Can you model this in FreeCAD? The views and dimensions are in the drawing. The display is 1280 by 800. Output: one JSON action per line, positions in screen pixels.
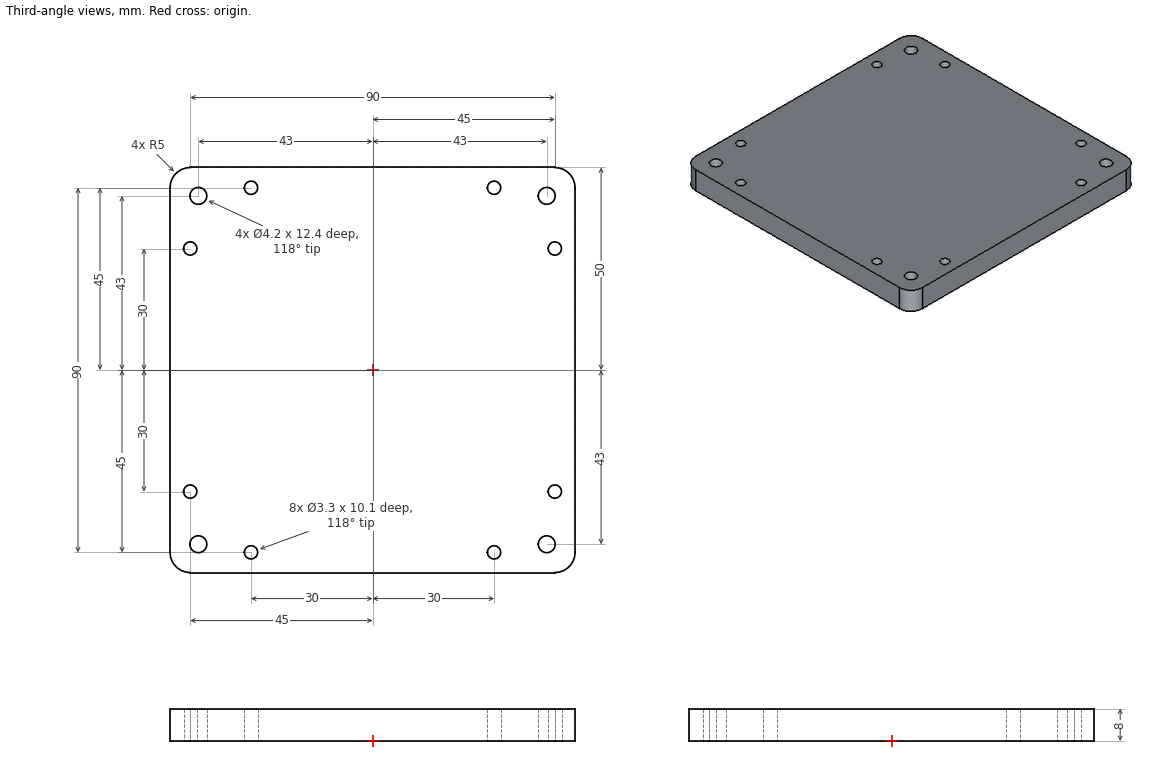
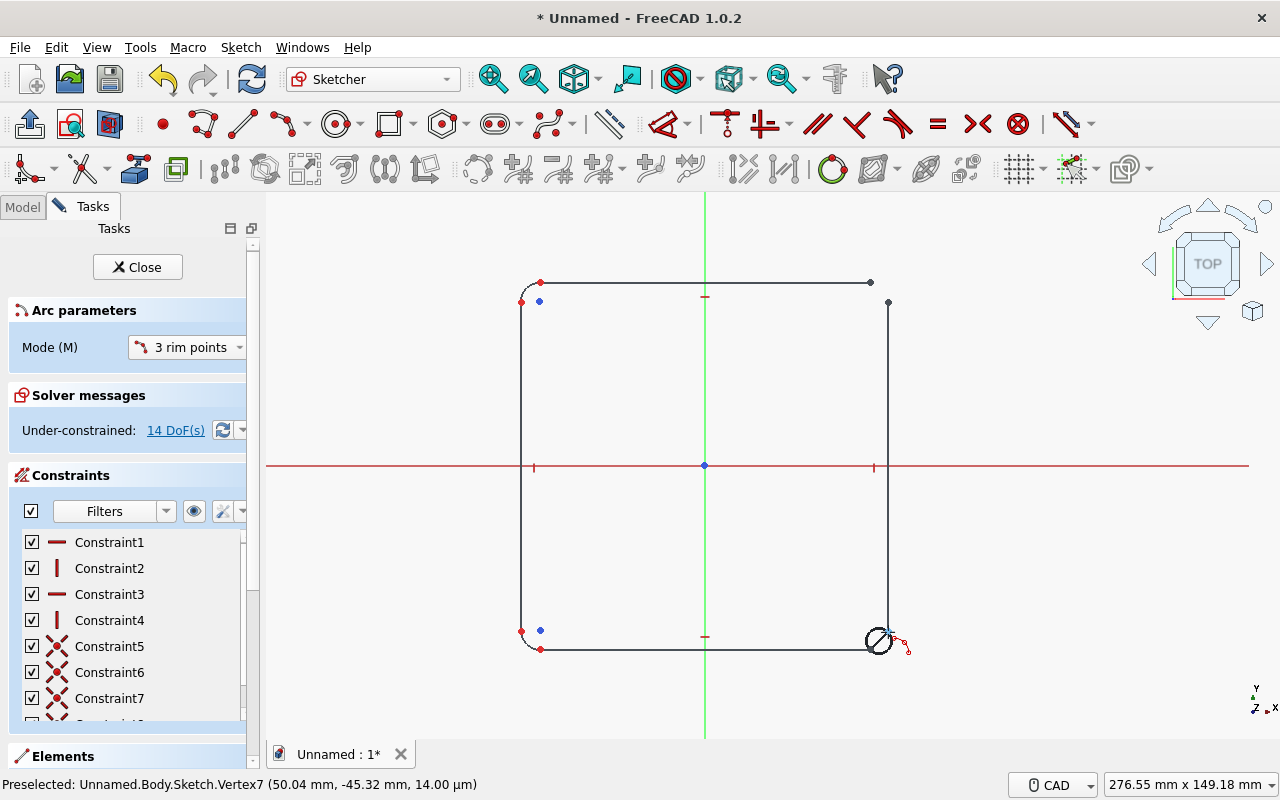
{"action": "scroll", "coordinate": [882, 644], "scroll_direction": "up", "scroll_amount": 6}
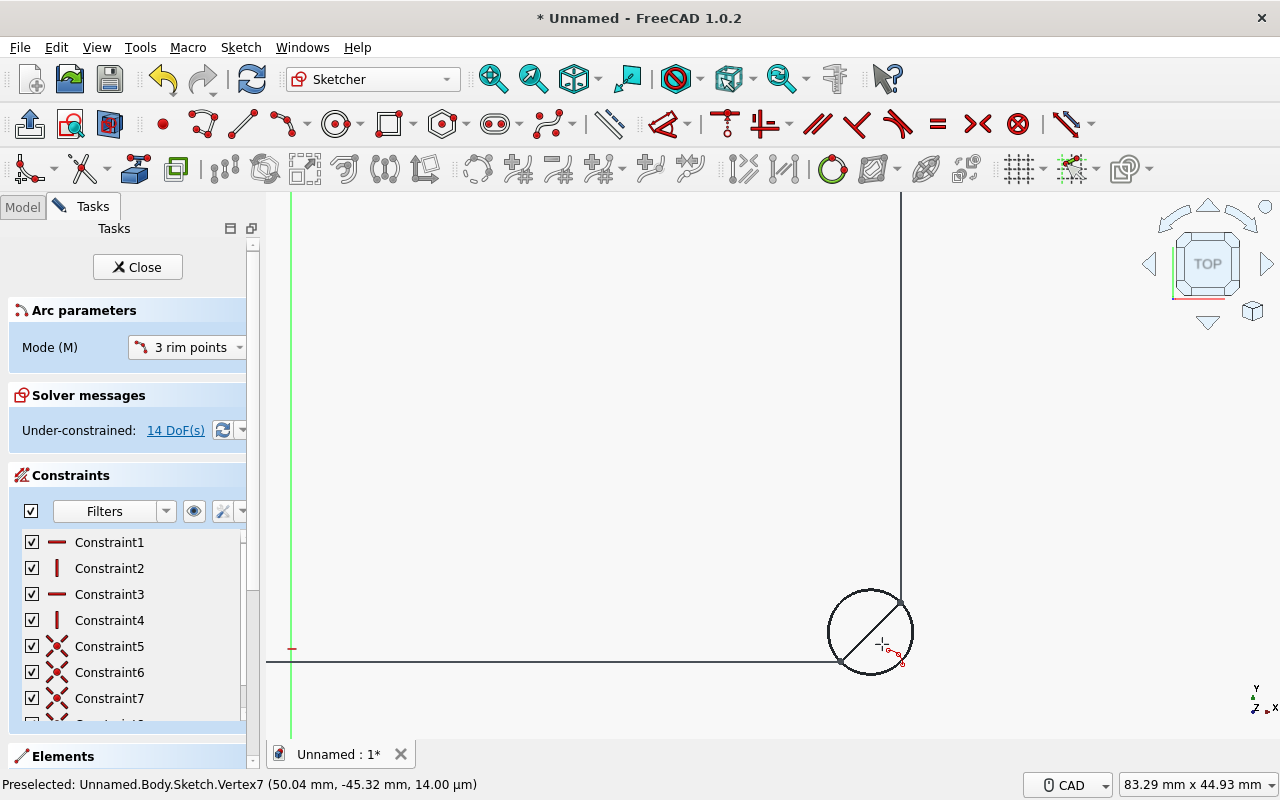
{"action": "left_click", "coordinate": [882, 641]}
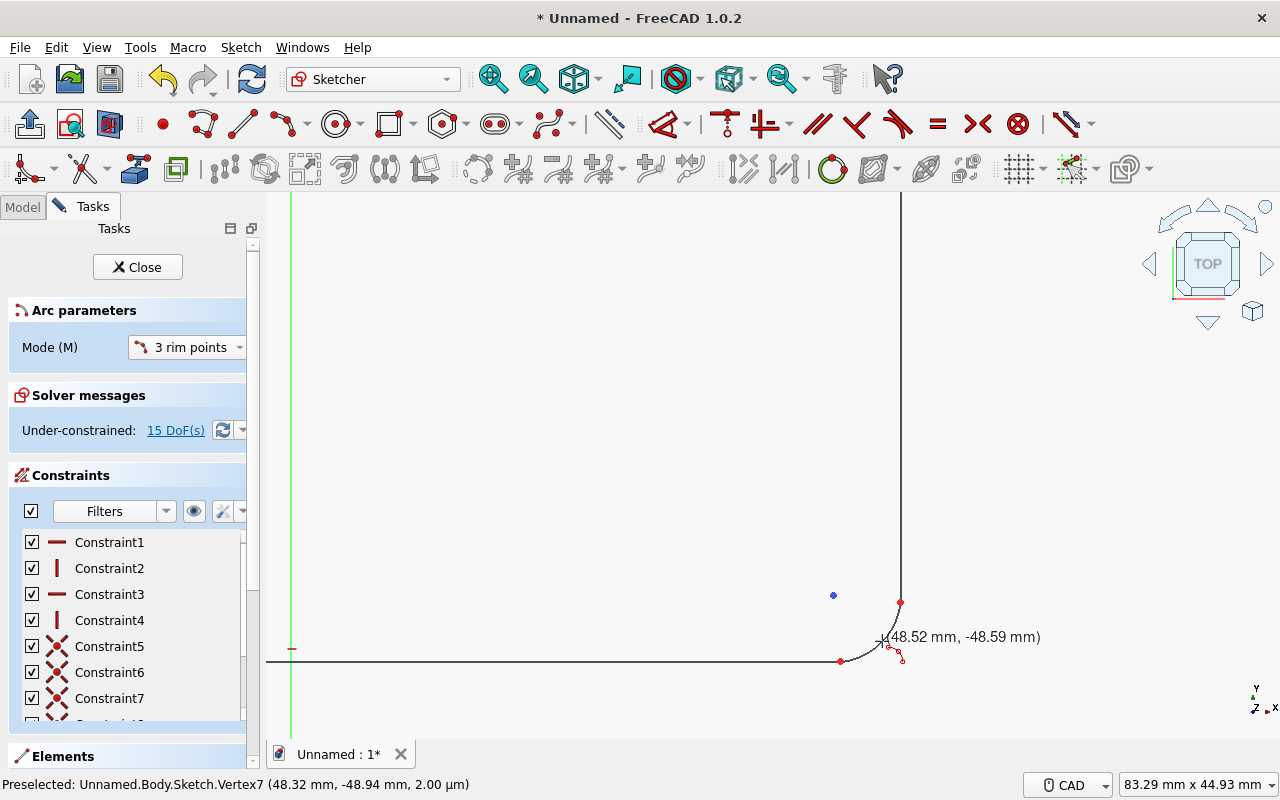
{"action": "scroll", "coordinate": [883, 644], "scroll_direction": "down", "scroll_amount": 6}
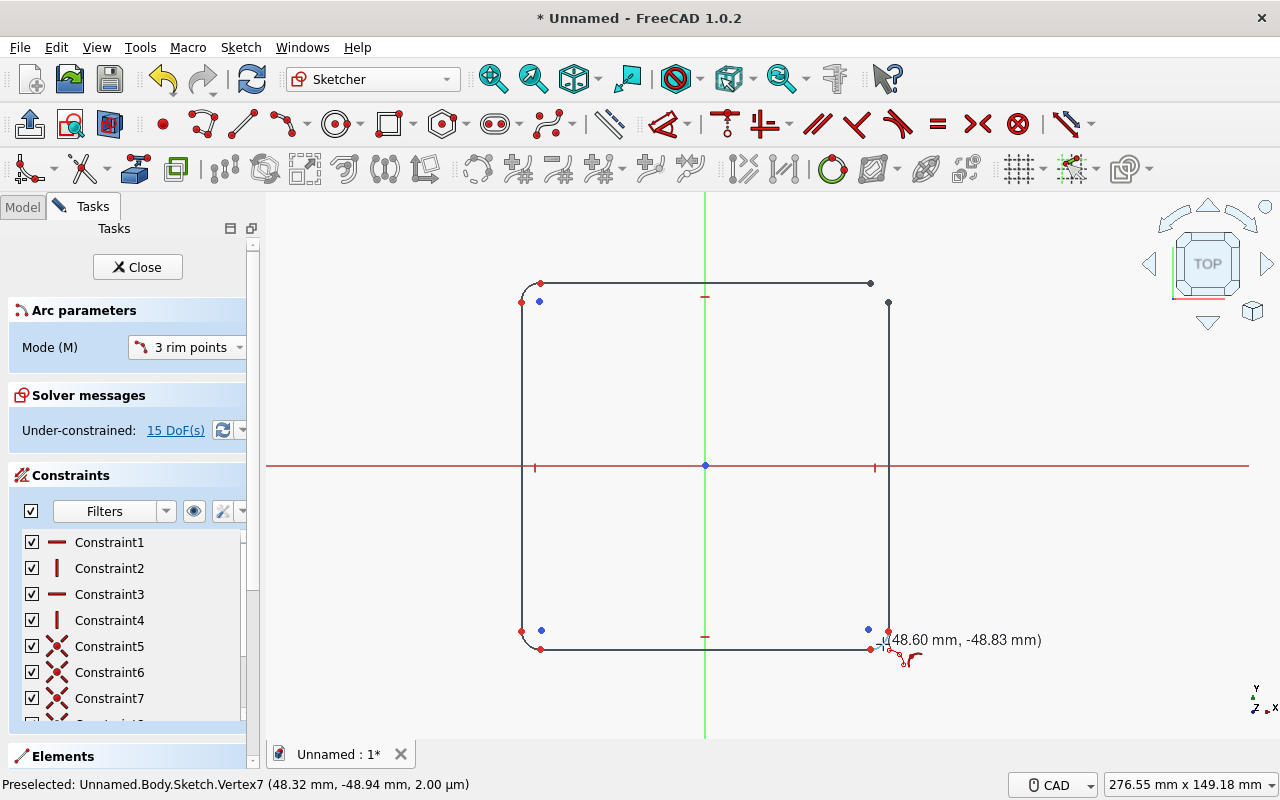
{"action": "left_click", "coordinate": [889, 302]}
{"action": "left_click", "coordinate": [871, 283]}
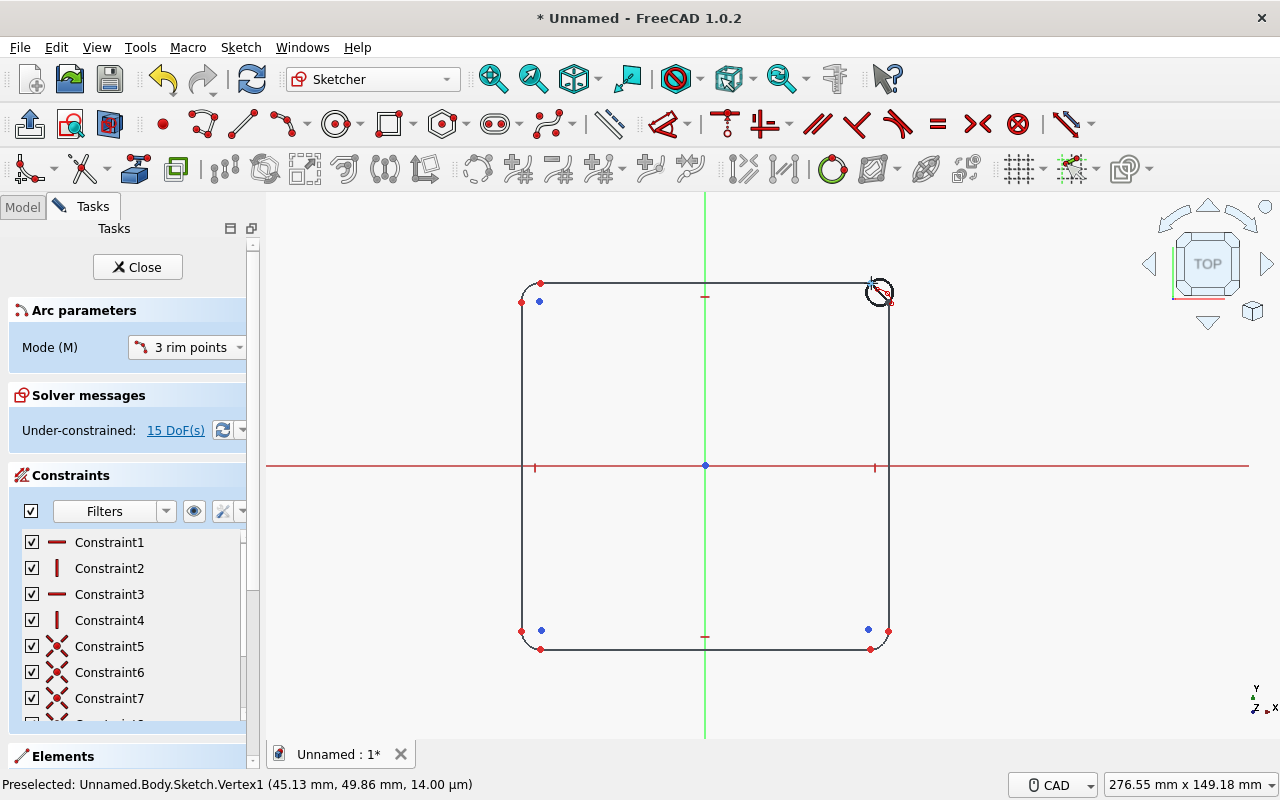
{"action": "scroll", "coordinate": [883, 288], "scroll_direction": "up", "scroll_amount": 6}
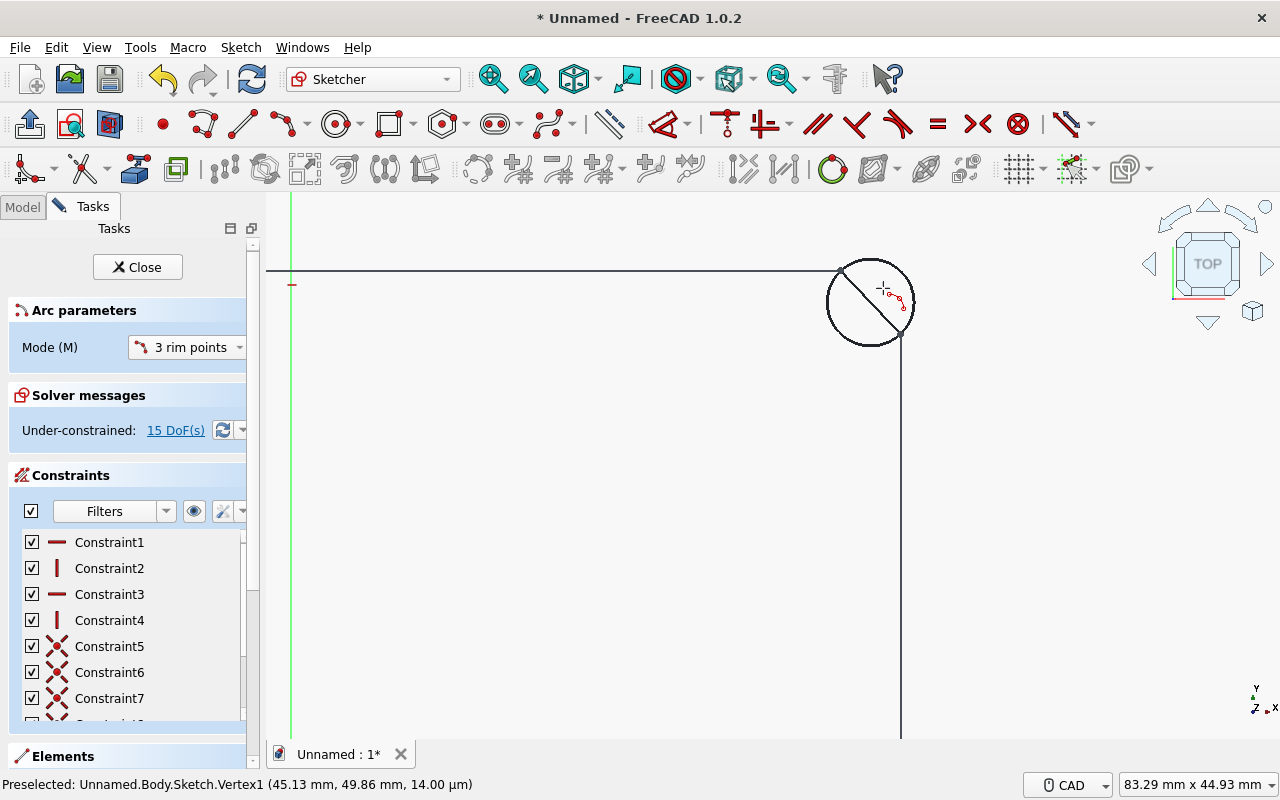
{"action": "left_click", "coordinate": [882, 287]}
{"action": "key", "text": "Escape"}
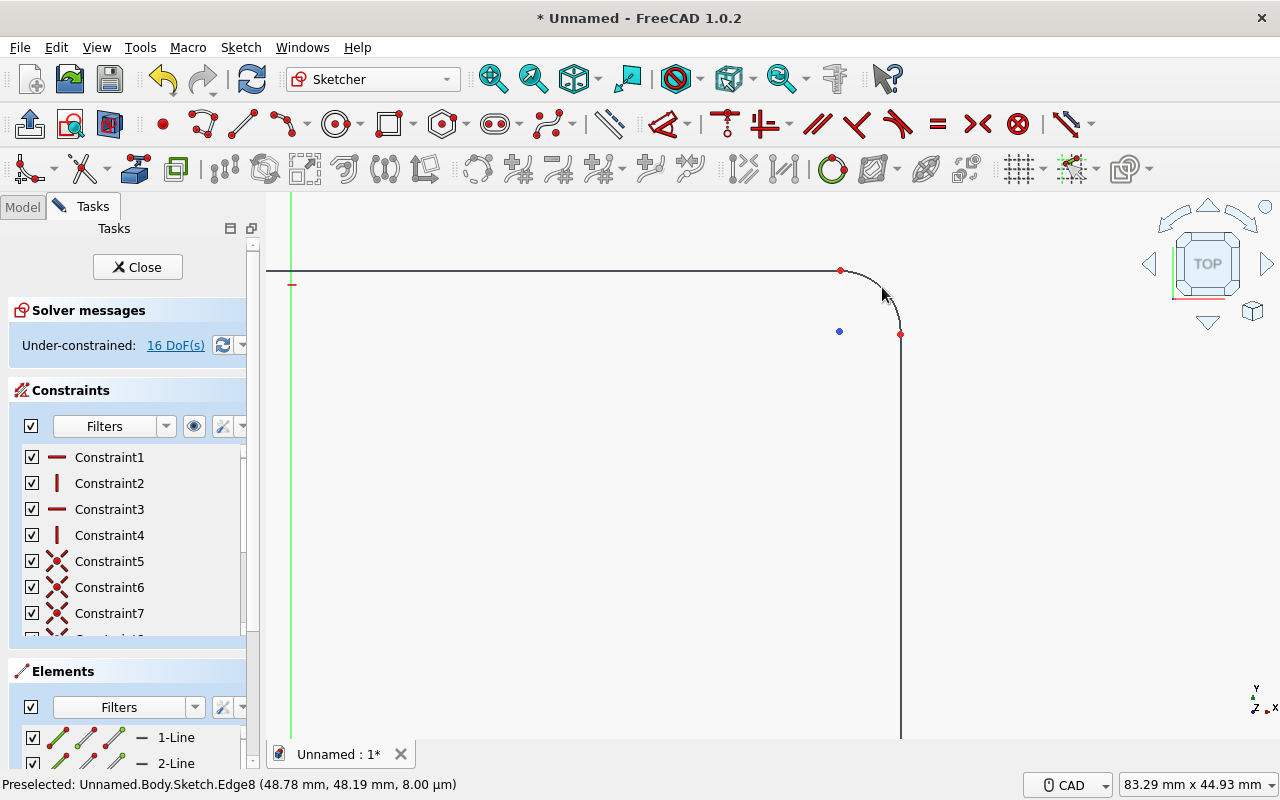
{"action": "left_click", "coordinate": [512, 271]}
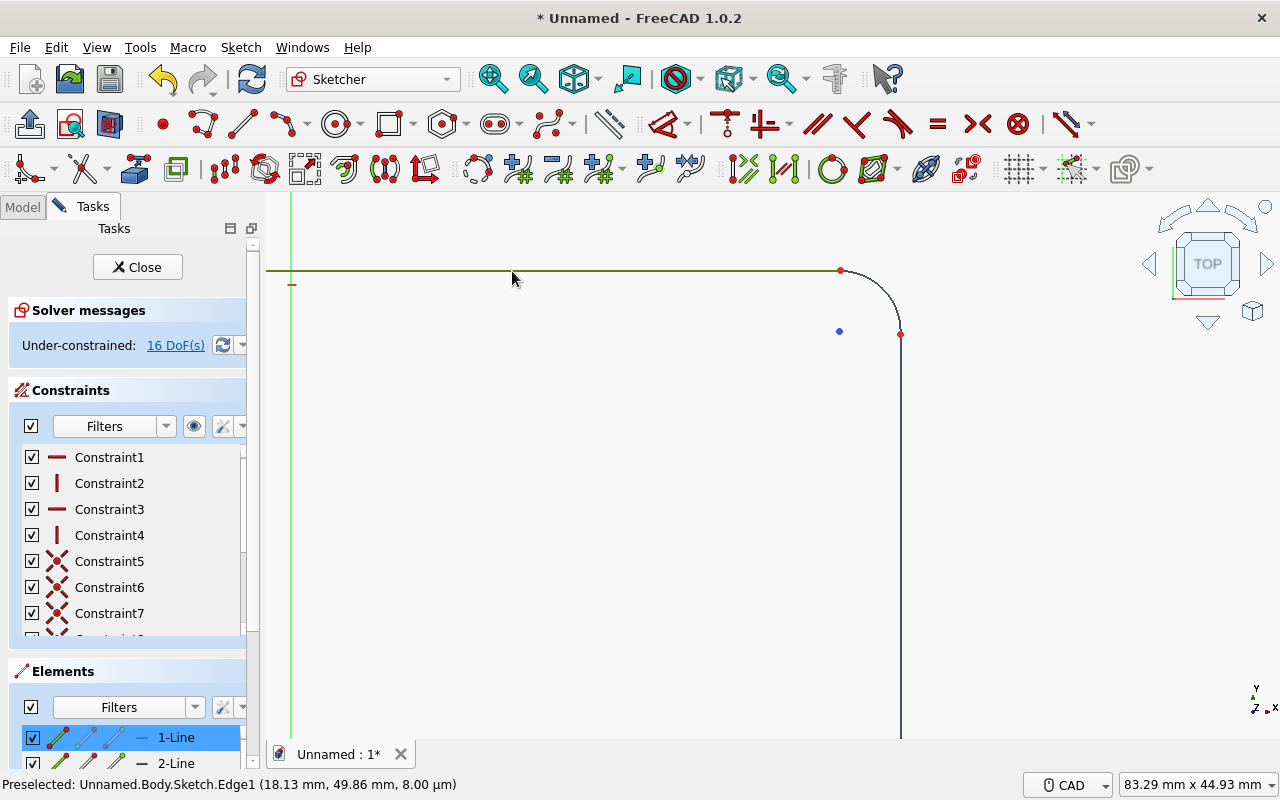
{"action": "scroll", "coordinate": [883, 288], "scroll_direction": "down", "scroll_amount": 6}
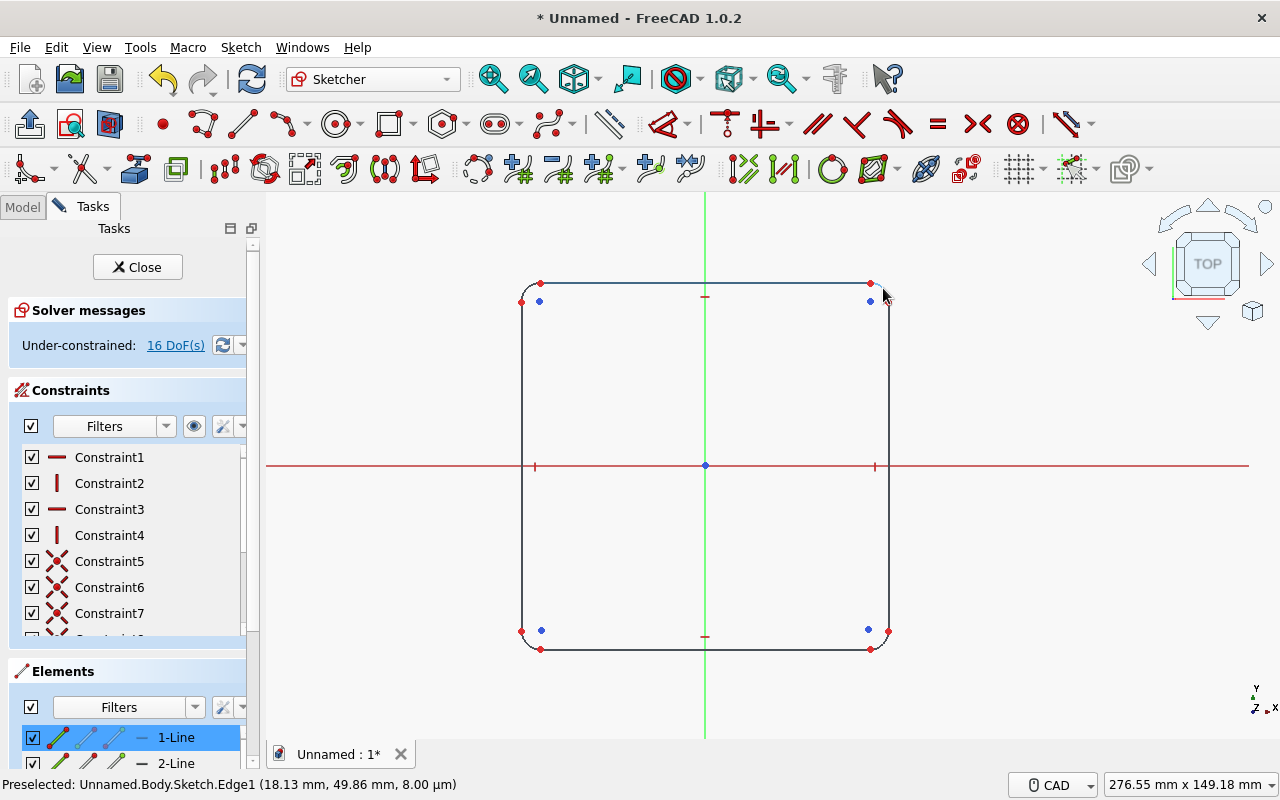
{"action": "scroll", "coordinate": [532, 285], "scroll_direction": "up", "scroll_amount": 3}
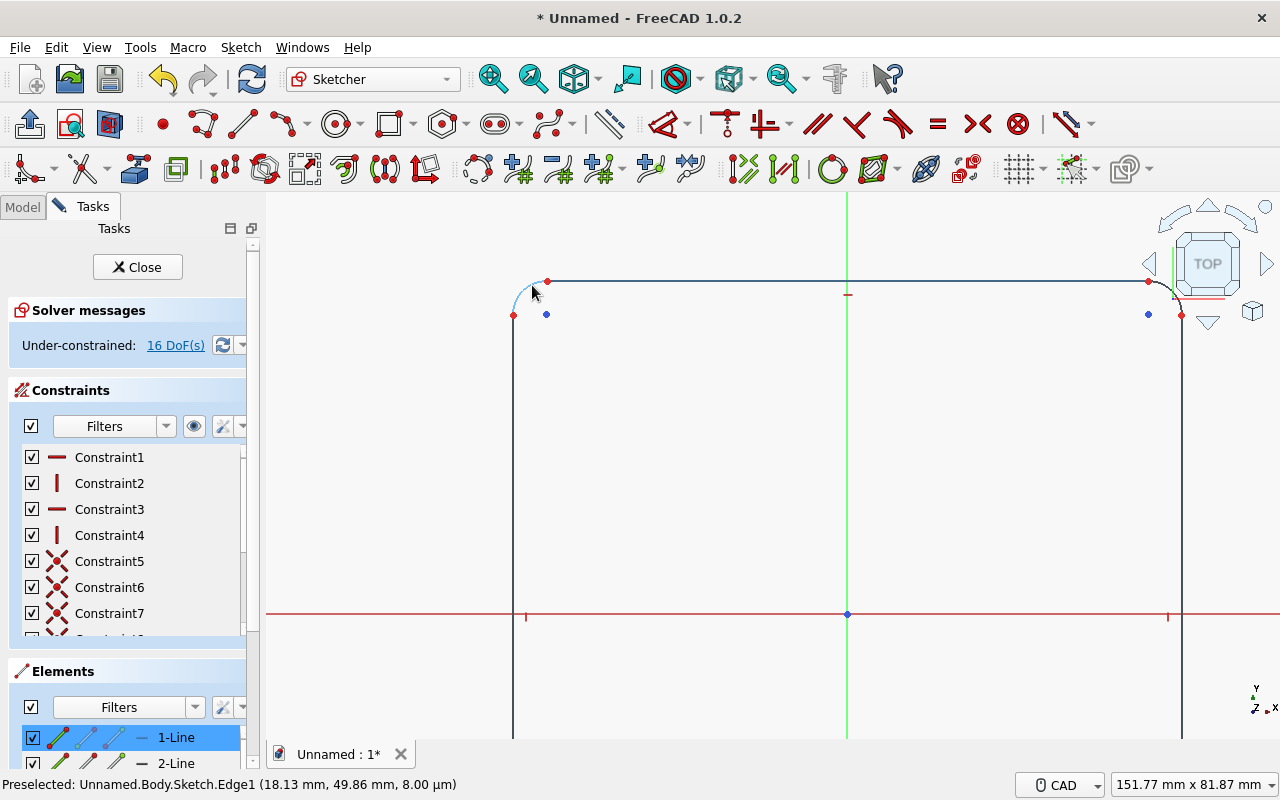
{"action": "left_click", "coordinate": [532, 285]}